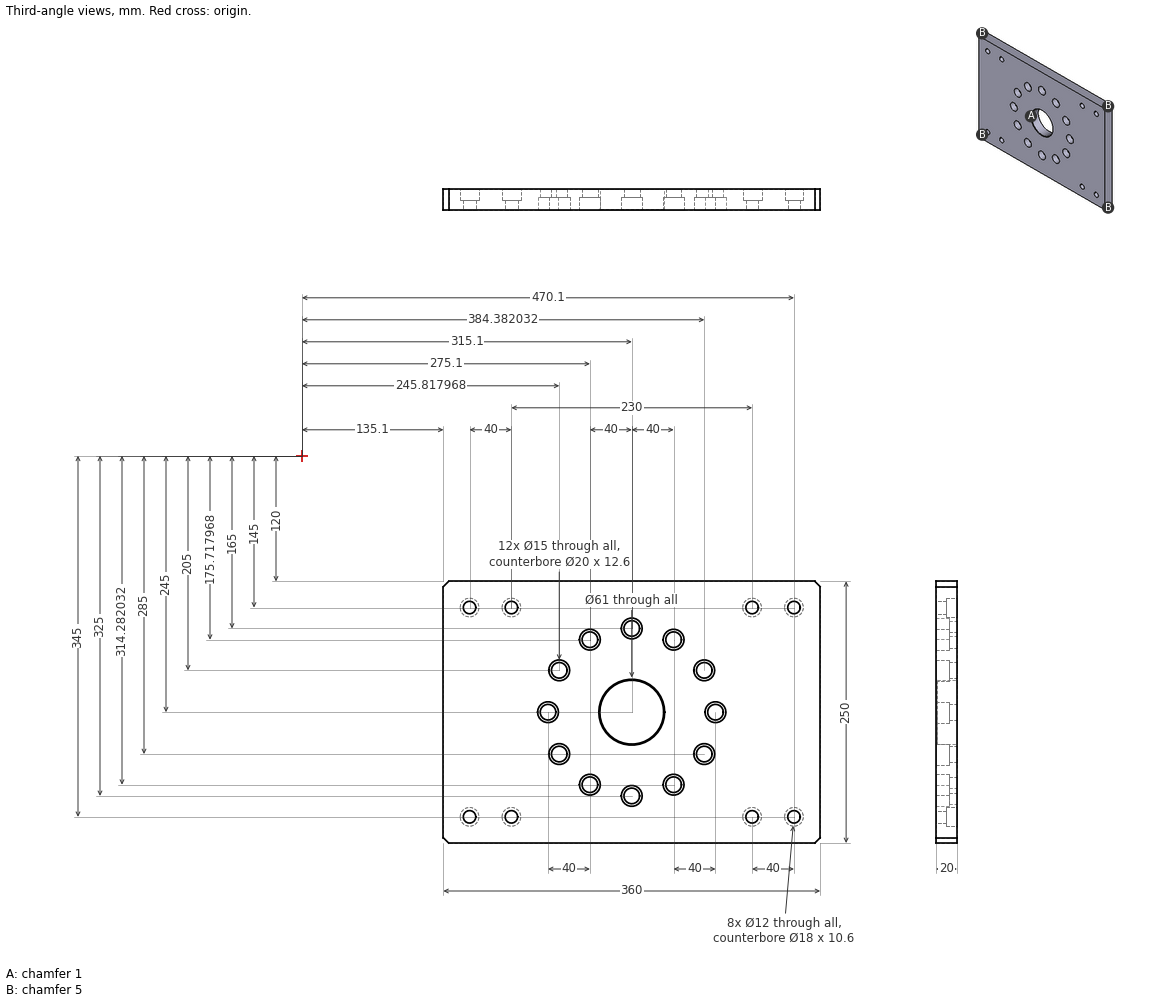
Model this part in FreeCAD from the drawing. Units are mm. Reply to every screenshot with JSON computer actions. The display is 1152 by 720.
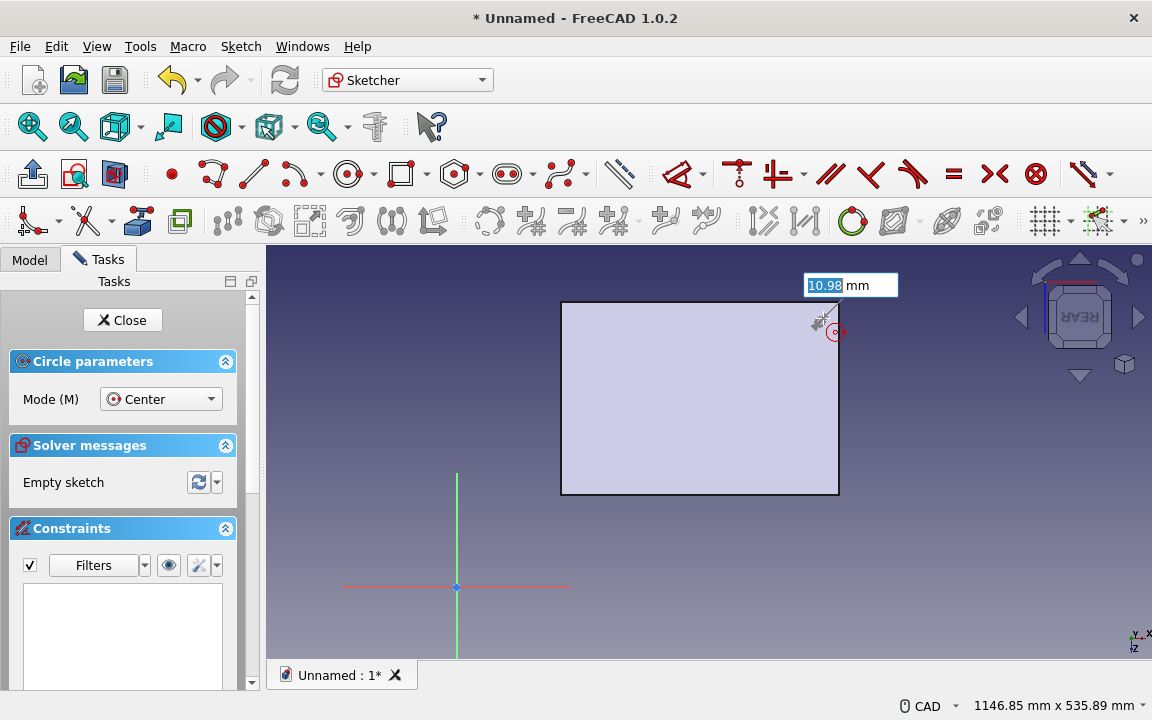
{"action": "type", "text": "12"}
{"action": "key", "text": "Return"}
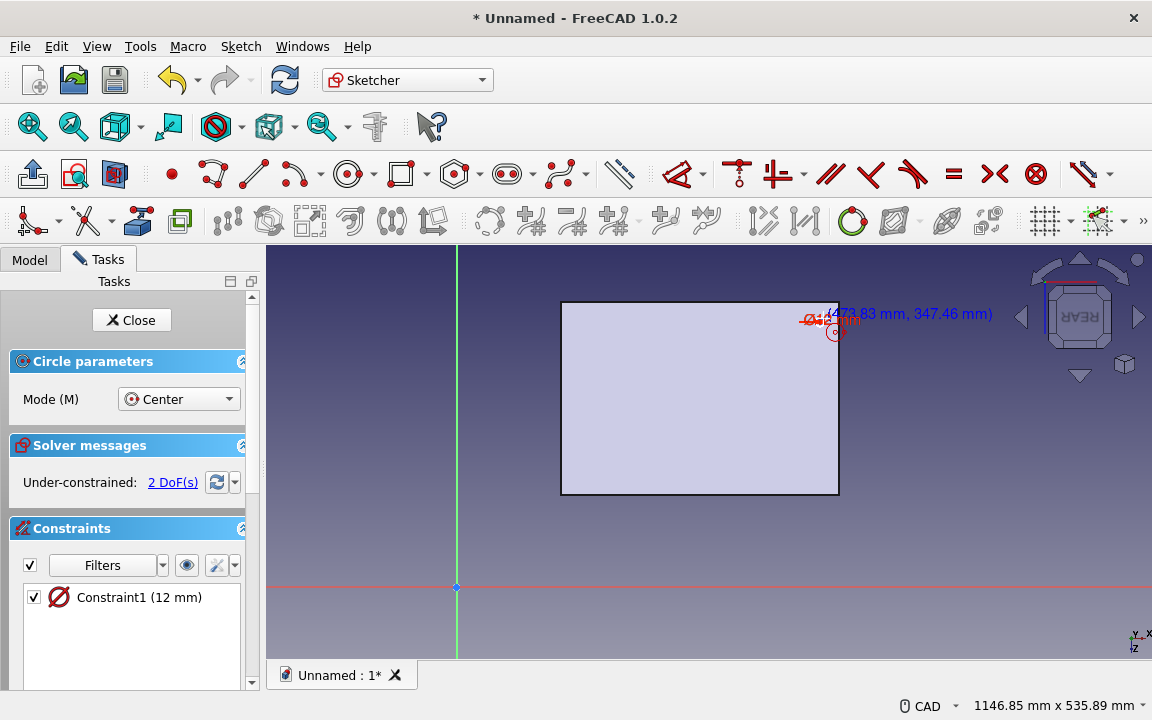
{"action": "scroll", "coordinate": [789, 321], "scroll_direction": "up", "scroll_amount": 8}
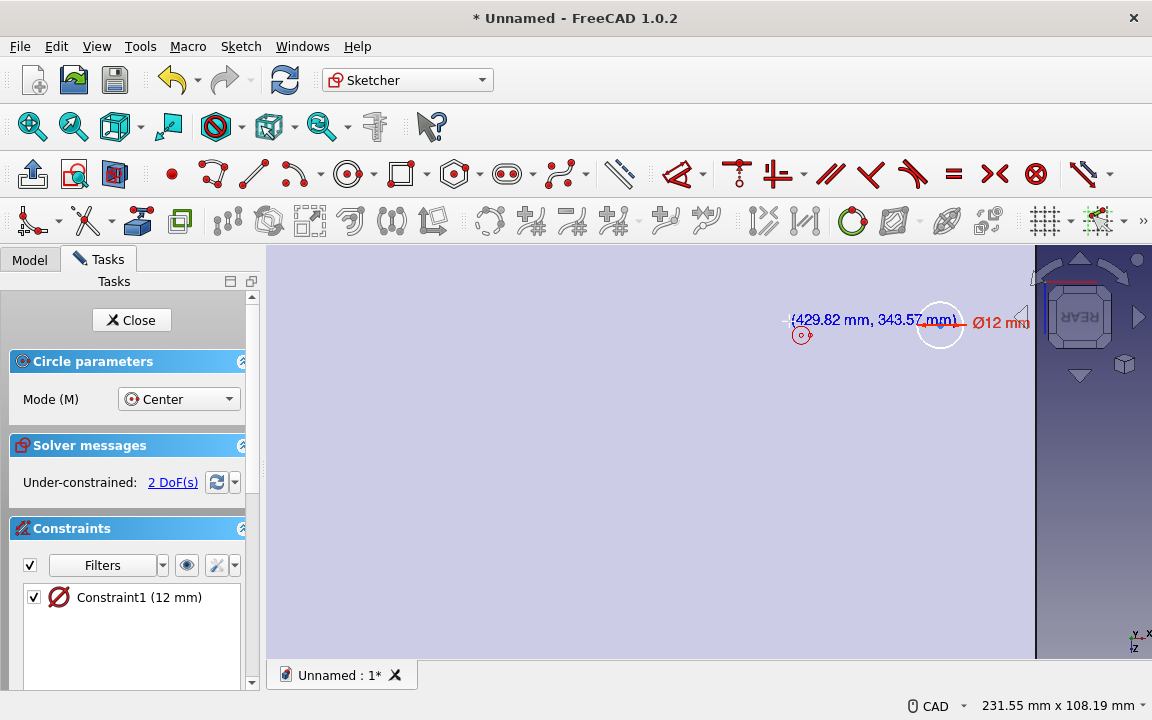
{"action": "scroll", "coordinate": [789, 321], "scroll_direction": "down", "scroll_amount": 8}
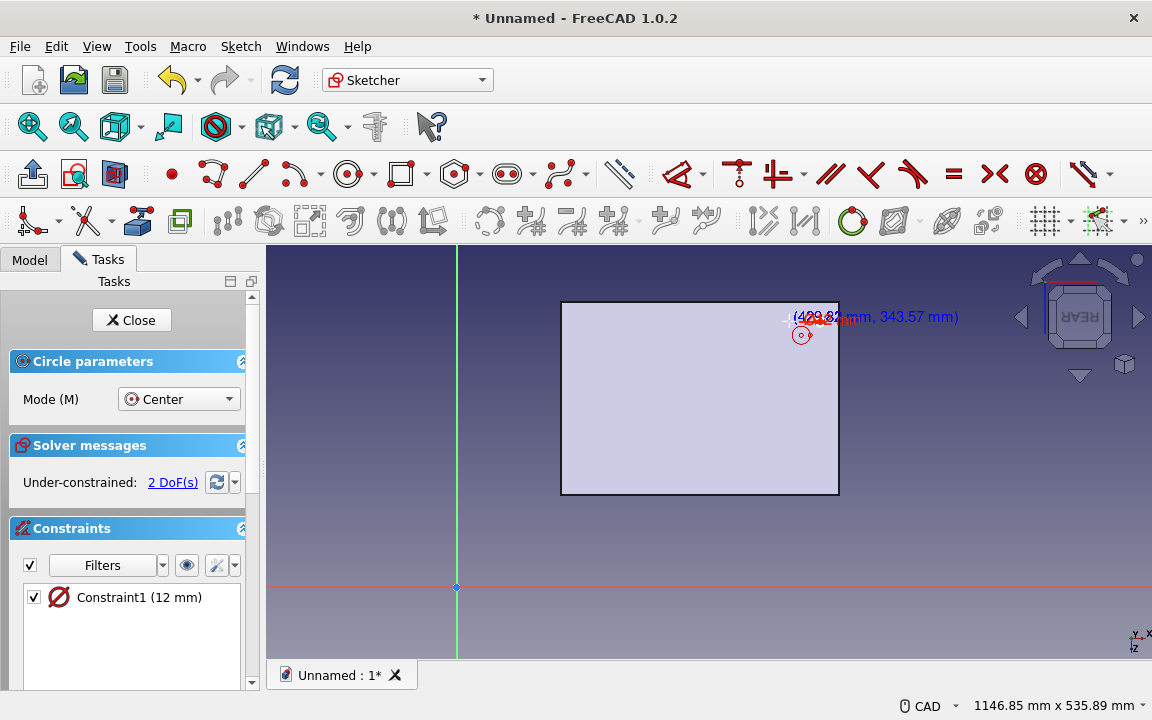
{"action": "left_click", "coordinate": [789, 321]}
{"action": "mouse_move", "coordinate": [792, 318]}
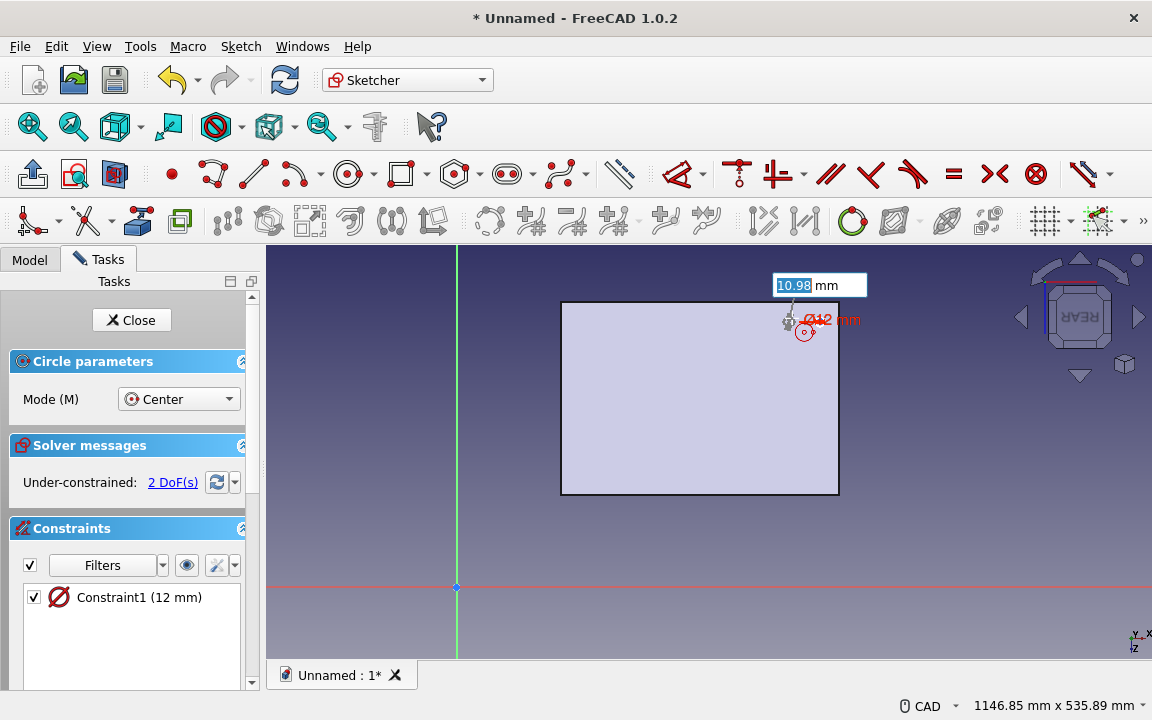
{"action": "type", "text": "12"}
{"action": "key", "text": "Return"}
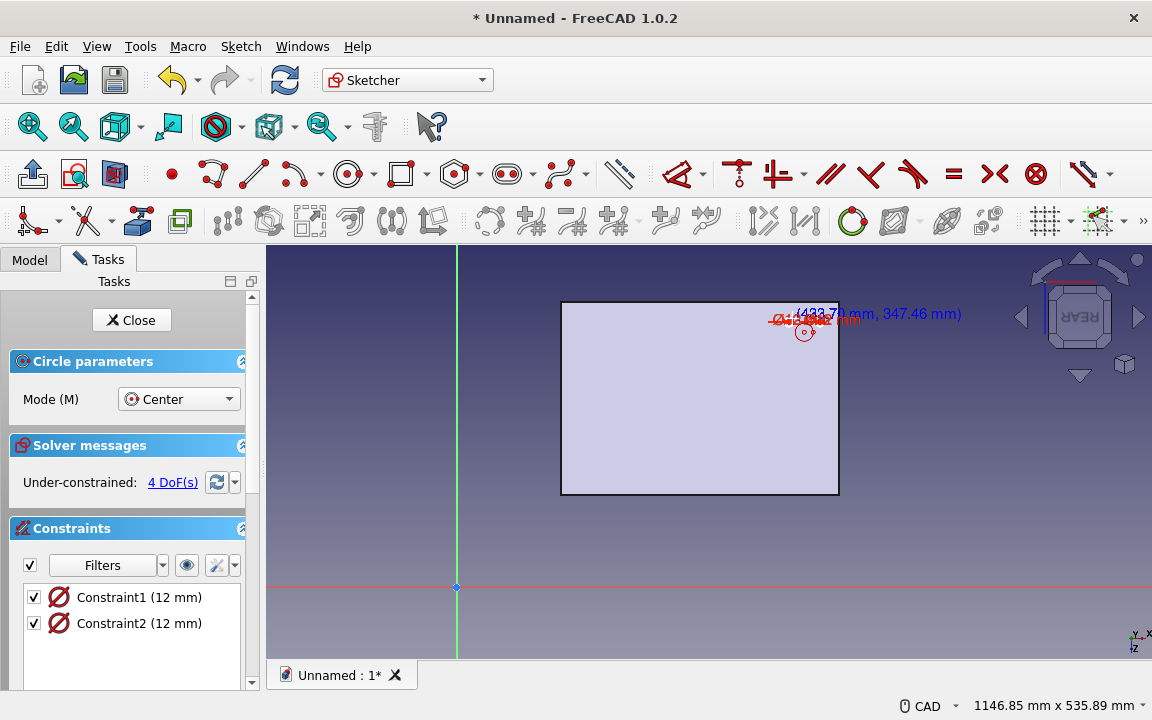
{"action": "scroll", "coordinate": [820, 475], "scroll_direction": "up", "scroll_amount": 8}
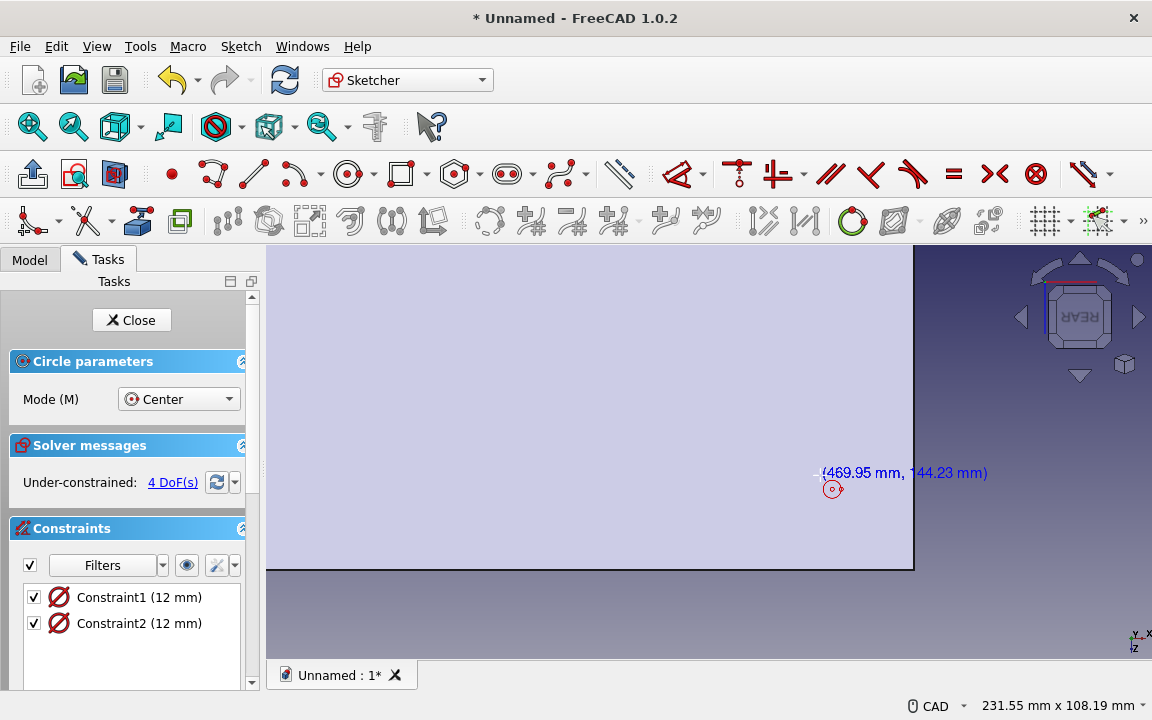
{"action": "scroll", "coordinate": [820, 476], "scroll_direction": "down", "scroll_amount": 8}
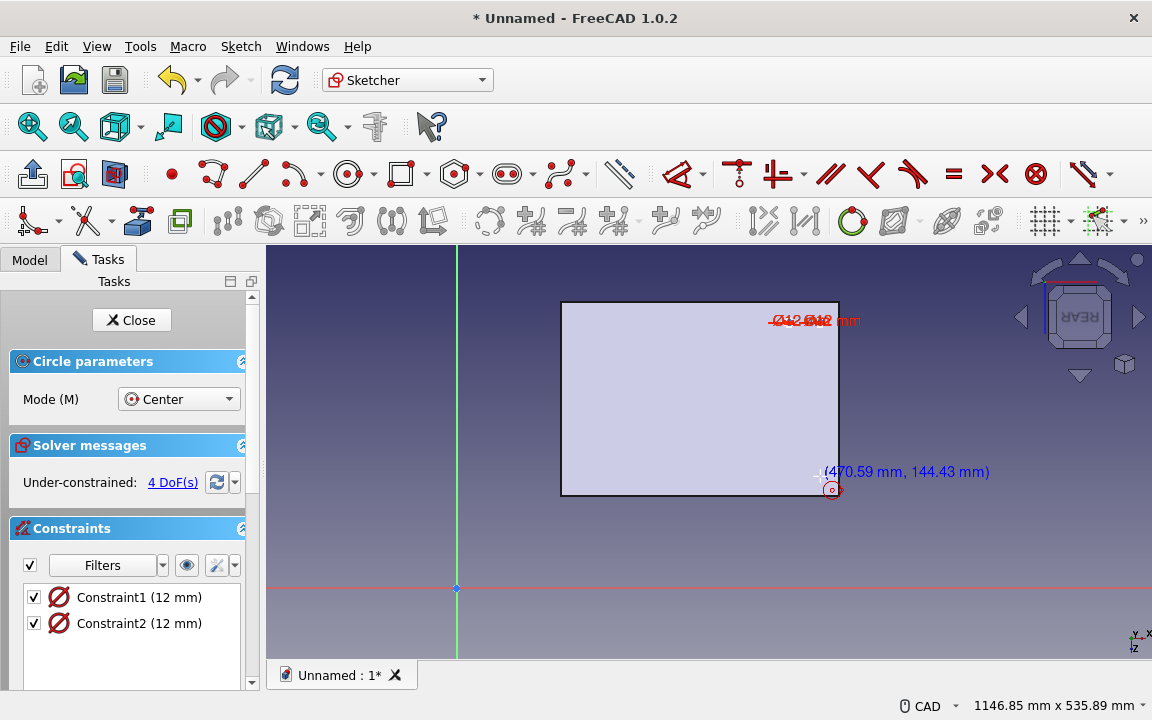
{"action": "left_click", "coordinate": [820, 476]}
{"action": "mouse_move", "coordinate": [823, 473]}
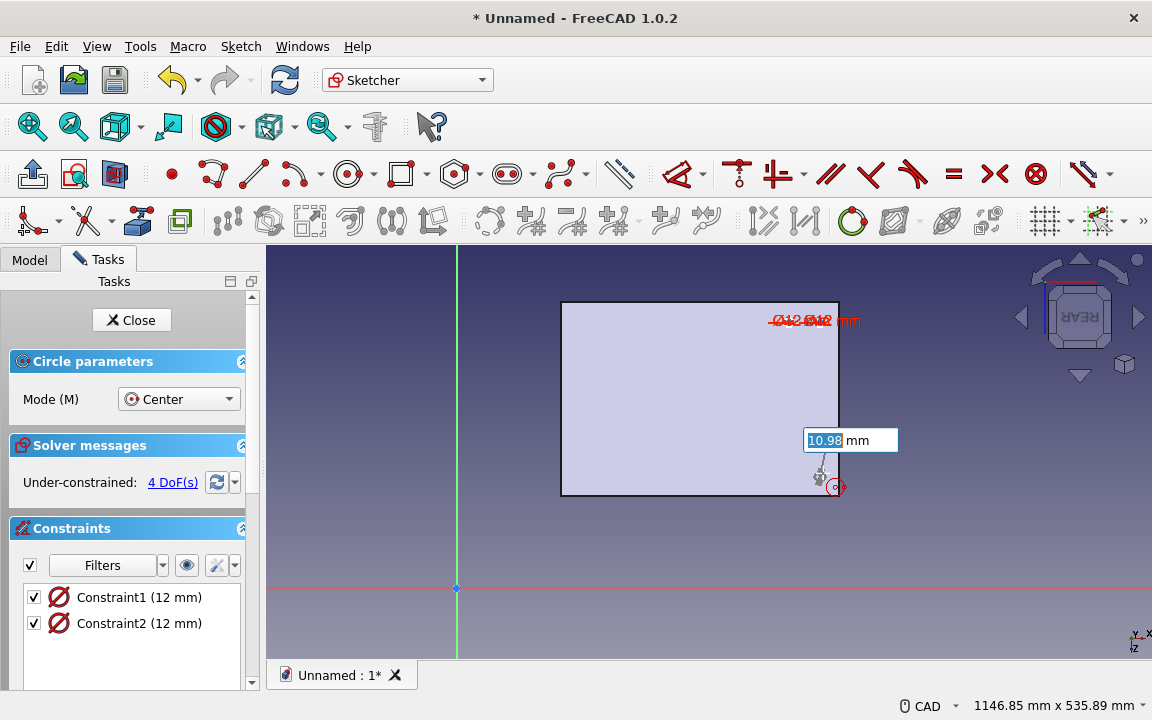
{"action": "type", "text": "12"}
{"action": "key", "text": "Return"}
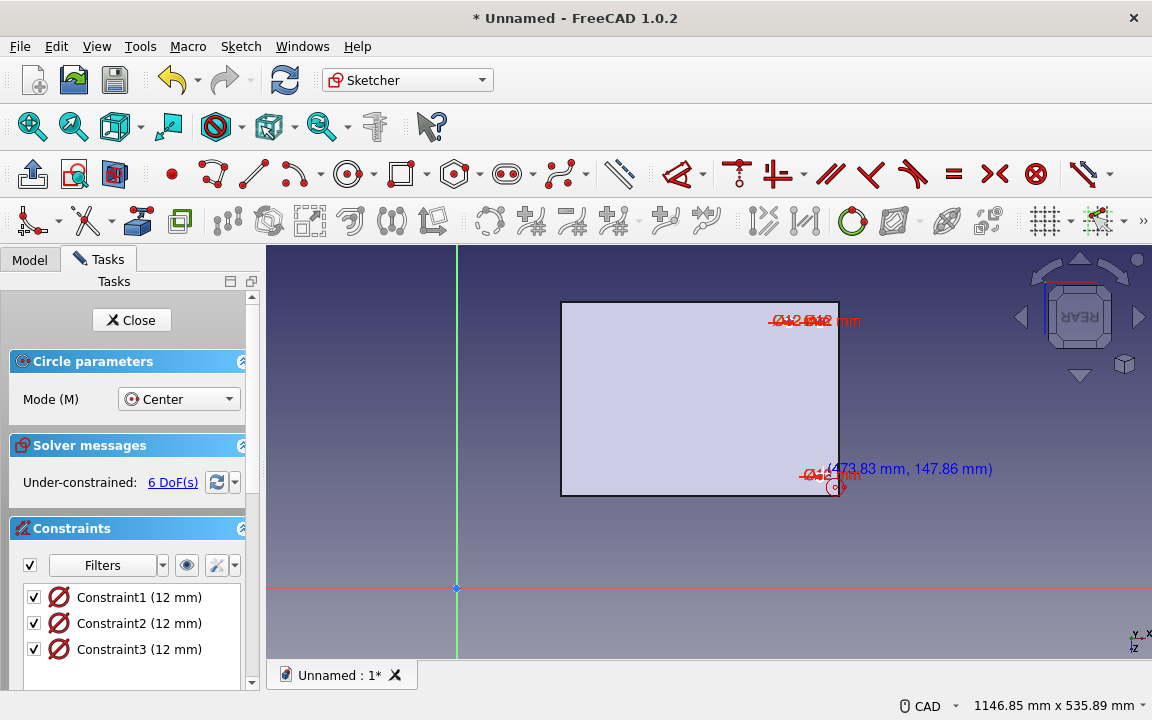
{"action": "scroll", "coordinate": [789, 476], "scroll_direction": "up", "scroll_amount": 8}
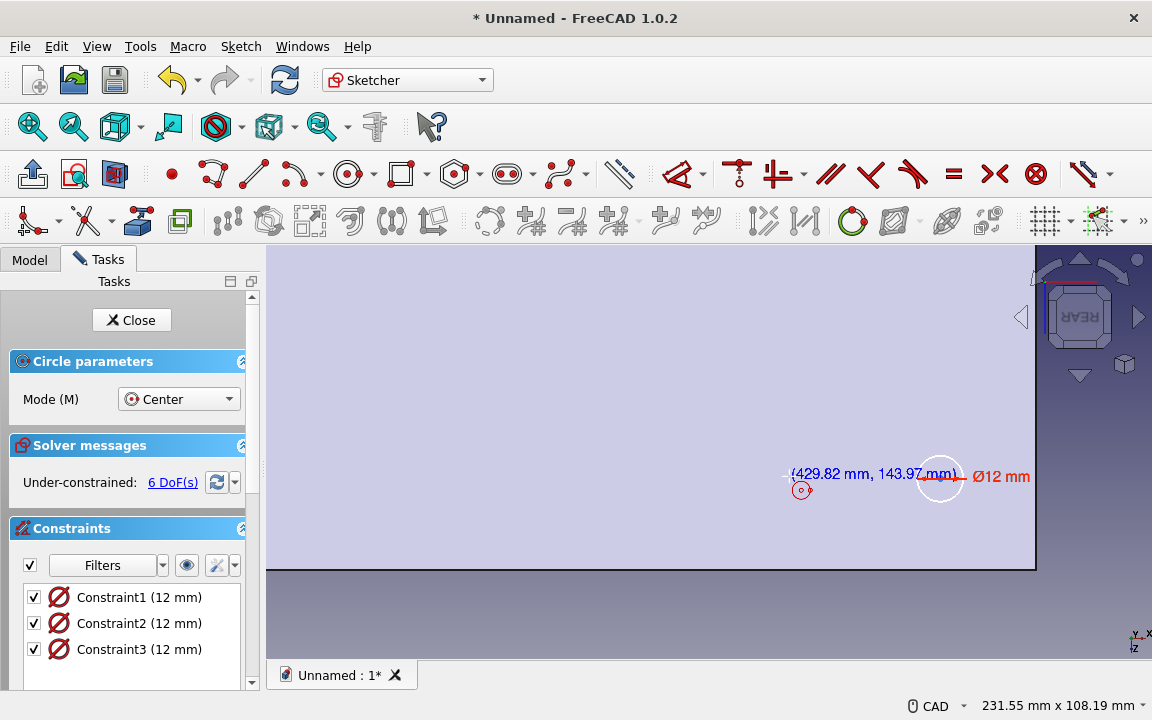
{"action": "scroll", "coordinate": [789, 476], "scroll_direction": "down", "scroll_amount": 8}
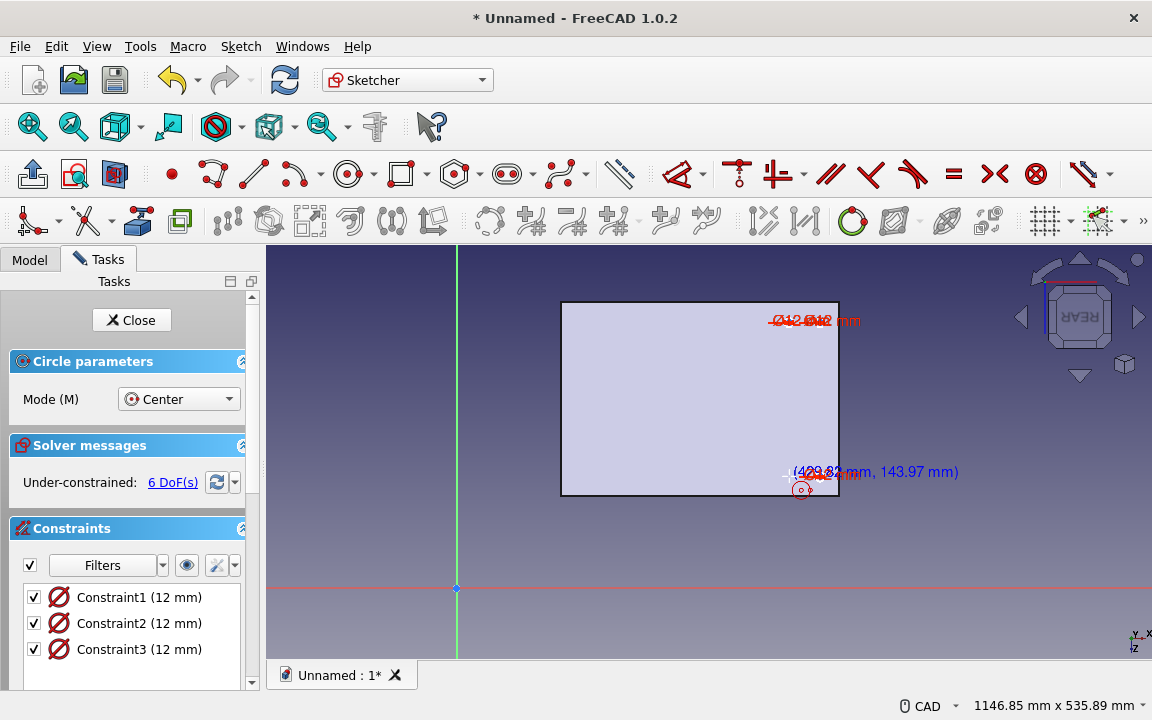
{"action": "left_click", "coordinate": [789, 476]}
{"action": "mouse_move", "coordinate": [792, 473]}